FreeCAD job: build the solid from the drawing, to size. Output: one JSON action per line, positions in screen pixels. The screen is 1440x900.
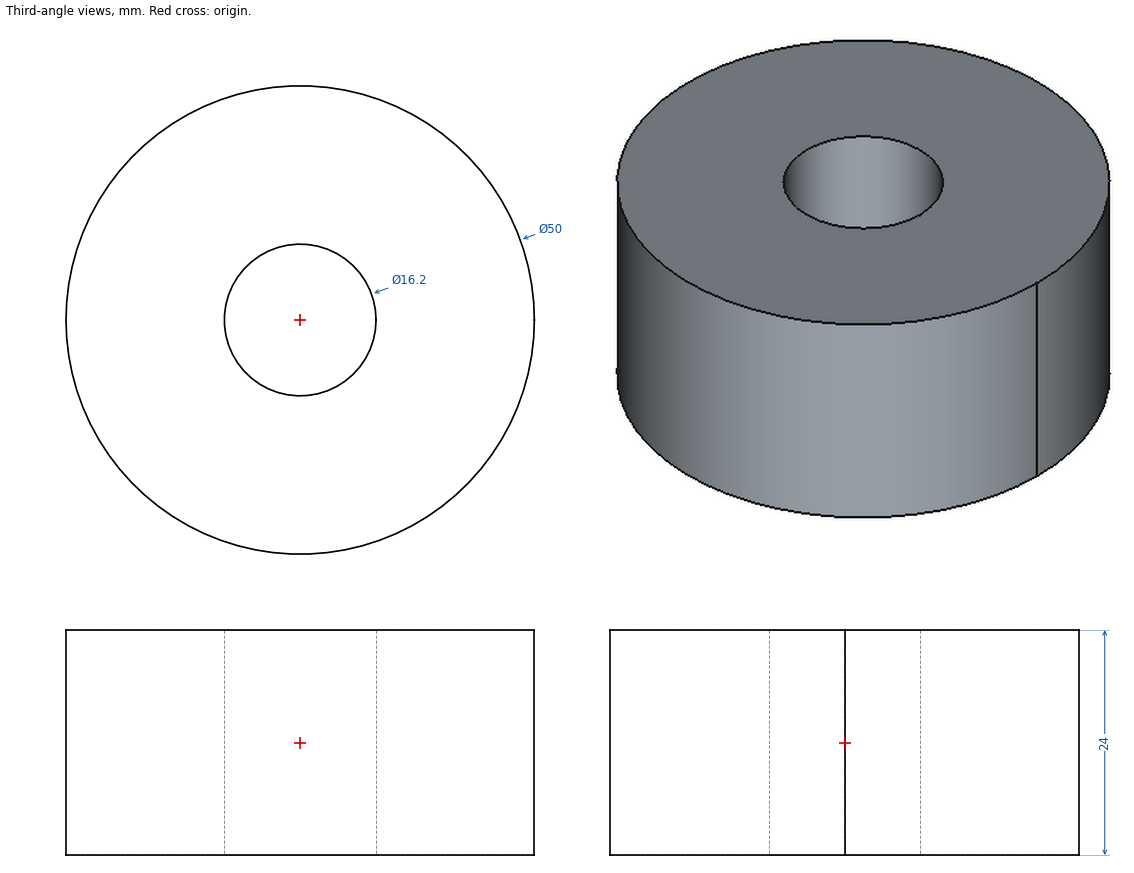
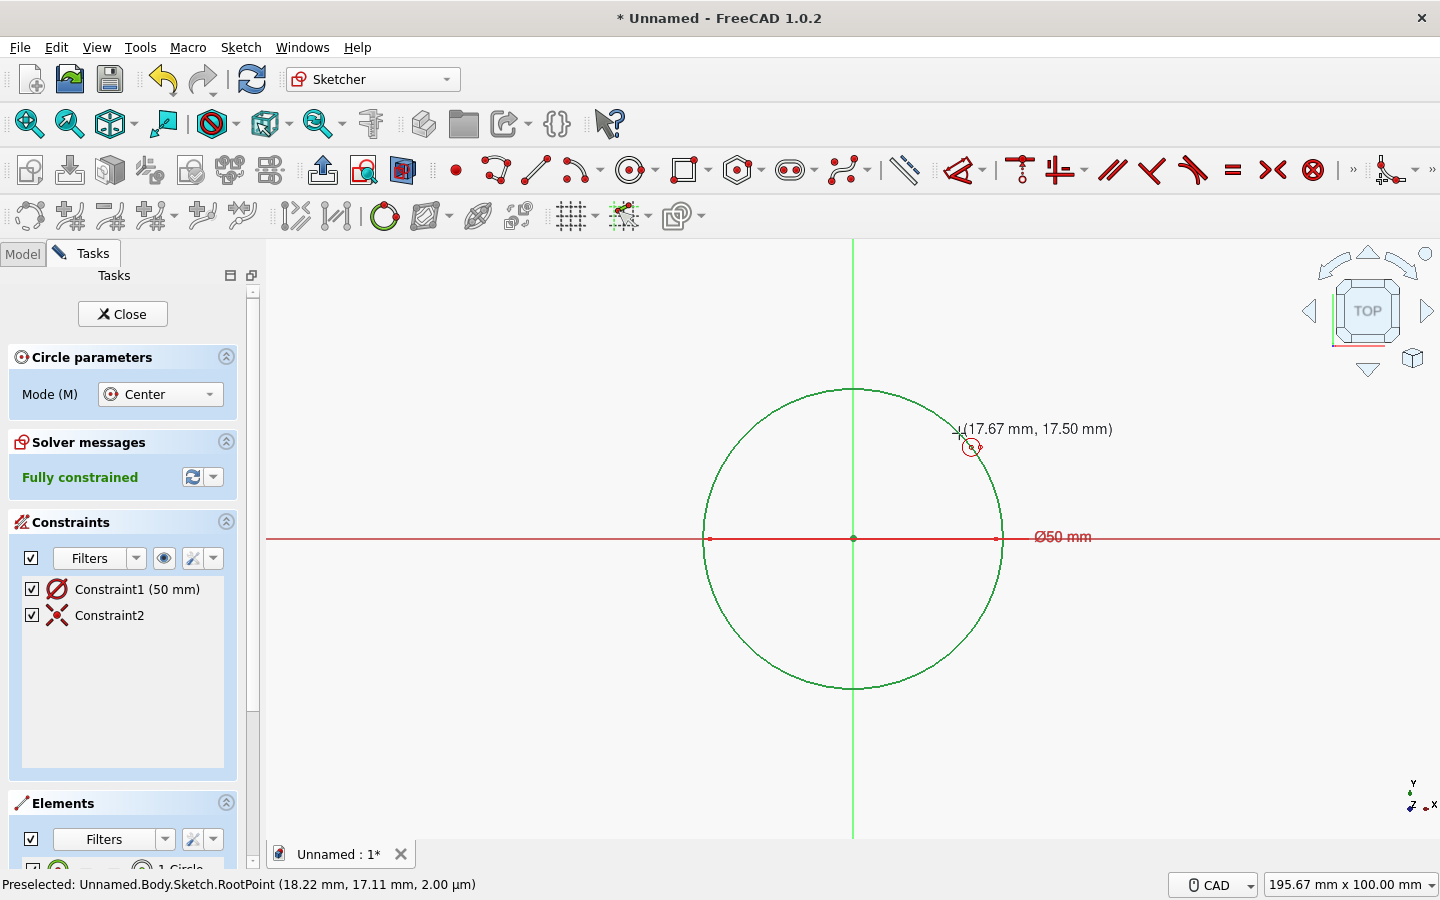
{"action": "left_click", "coordinate": [853, 539]}
{"action": "mouse_move", "coordinate": [887, 505]}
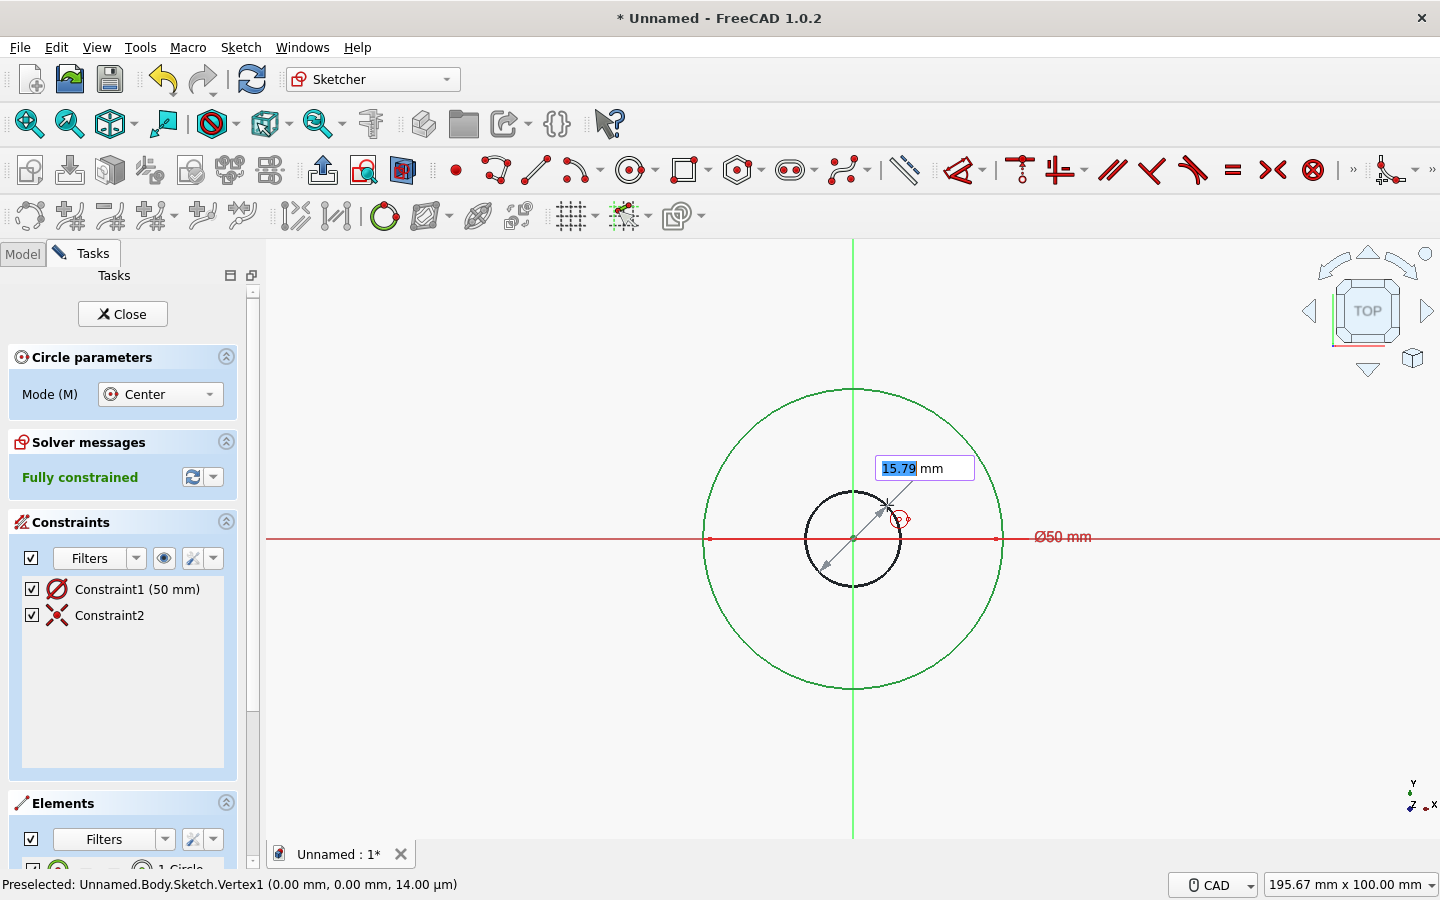
{"action": "type", "text": "16.2"}
{"action": "key", "text": "Return"}
{"action": "key", "text": "Escape"}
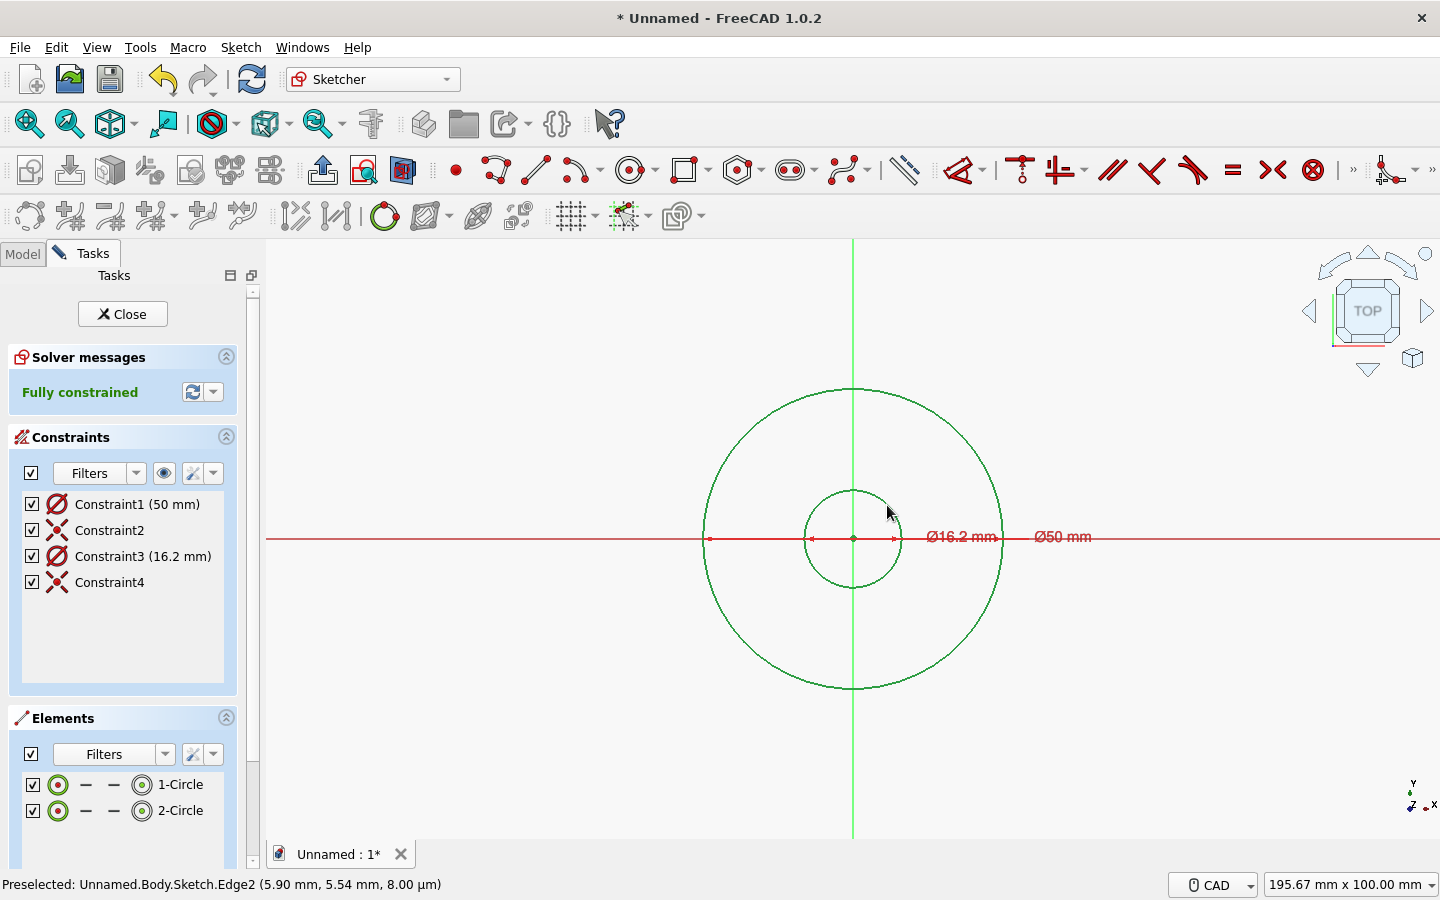
{"action": "left_click", "coordinate": [123, 314]}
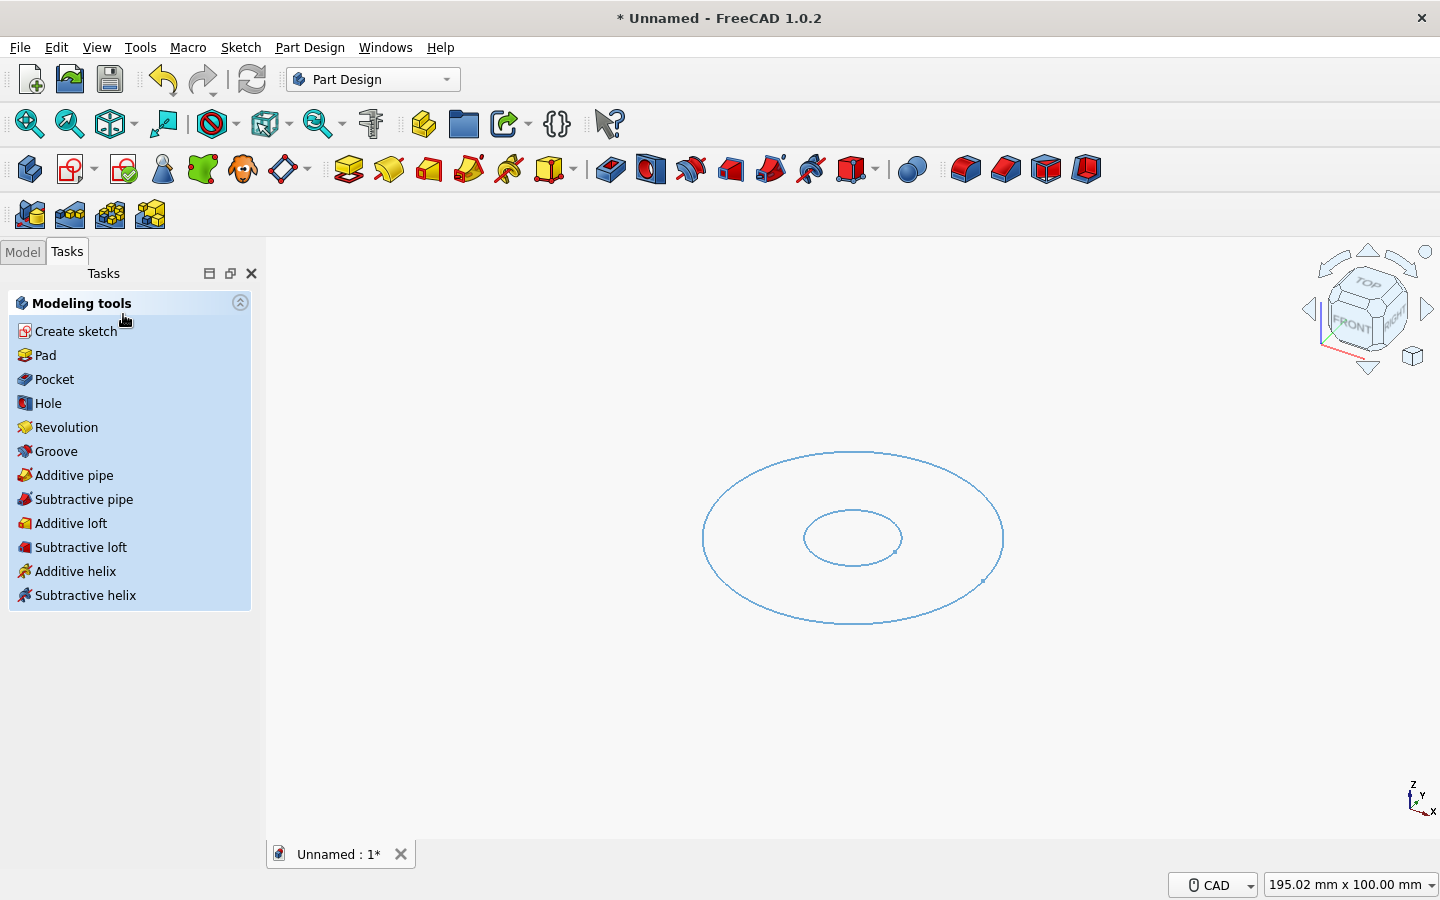
{"action": "left_click", "coordinate": [350, 170]}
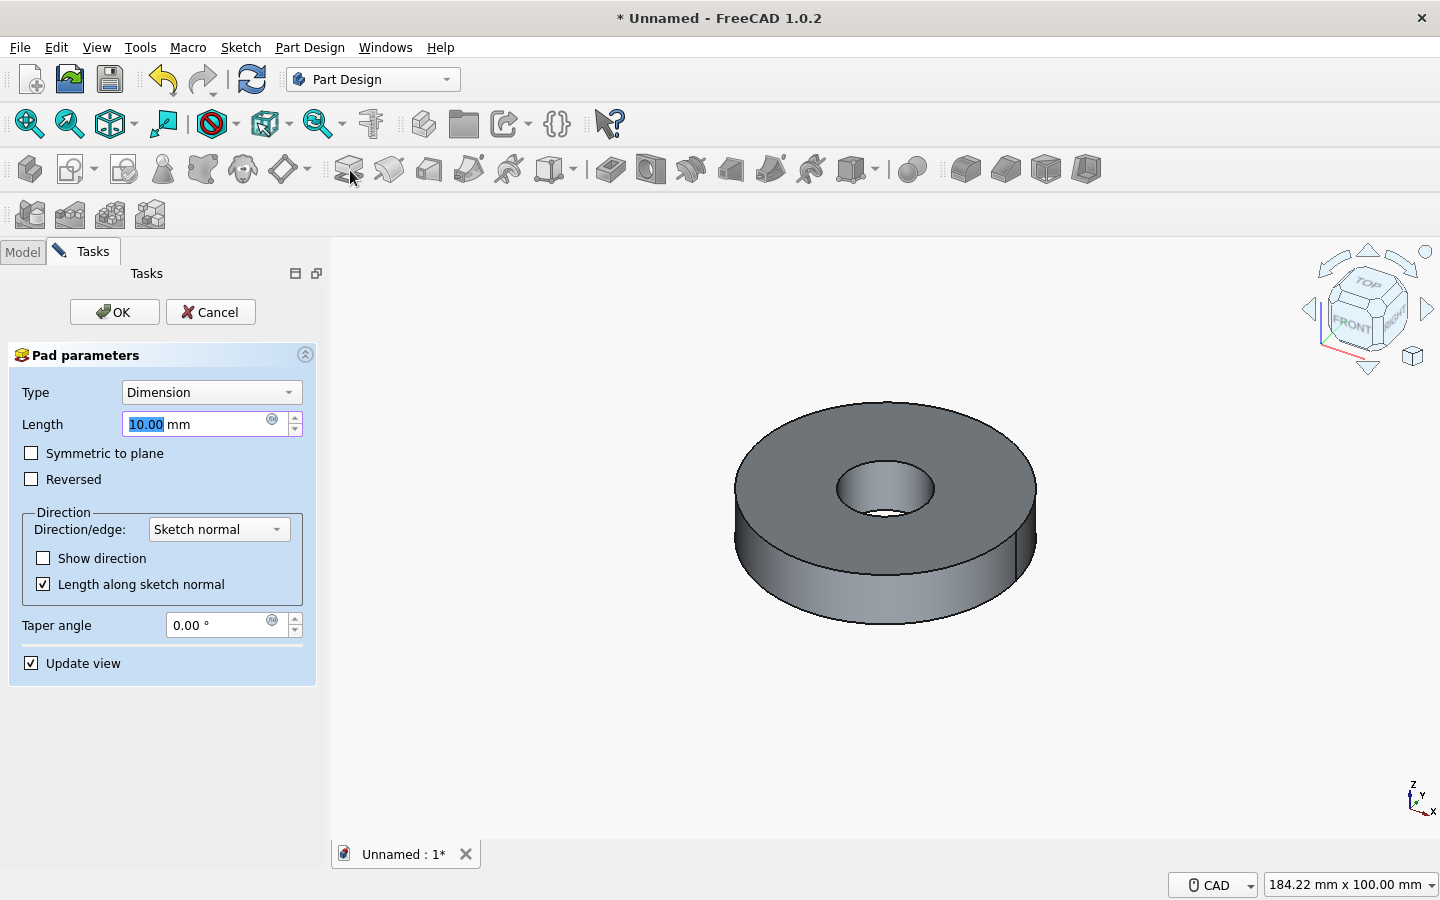
{"action": "type", "text": "24"}
{"action": "key", "text": "Tab"}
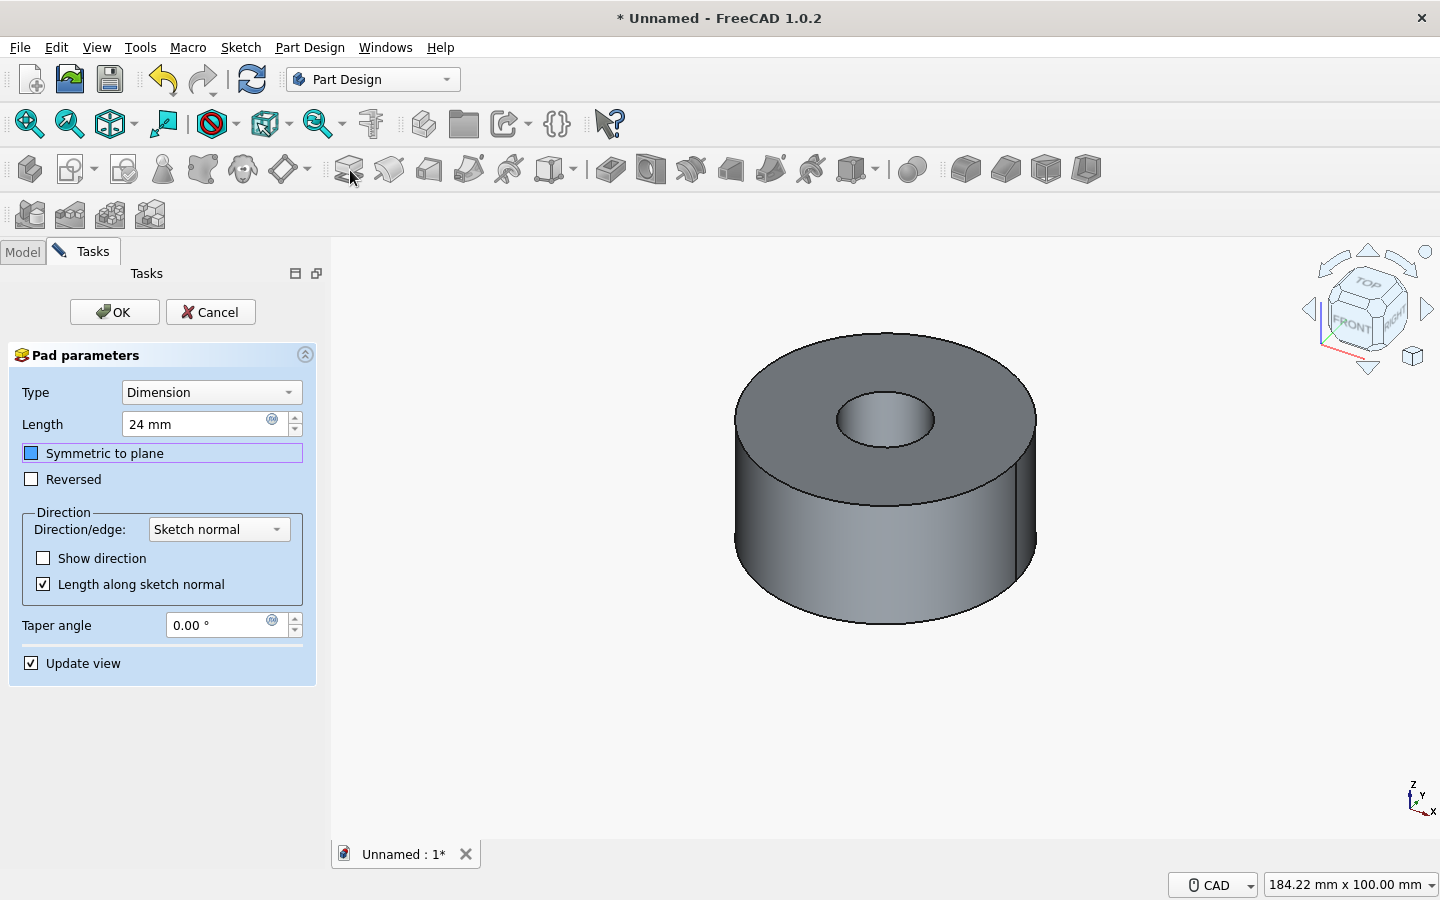
{"action": "left_click", "coordinate": [30, 453]}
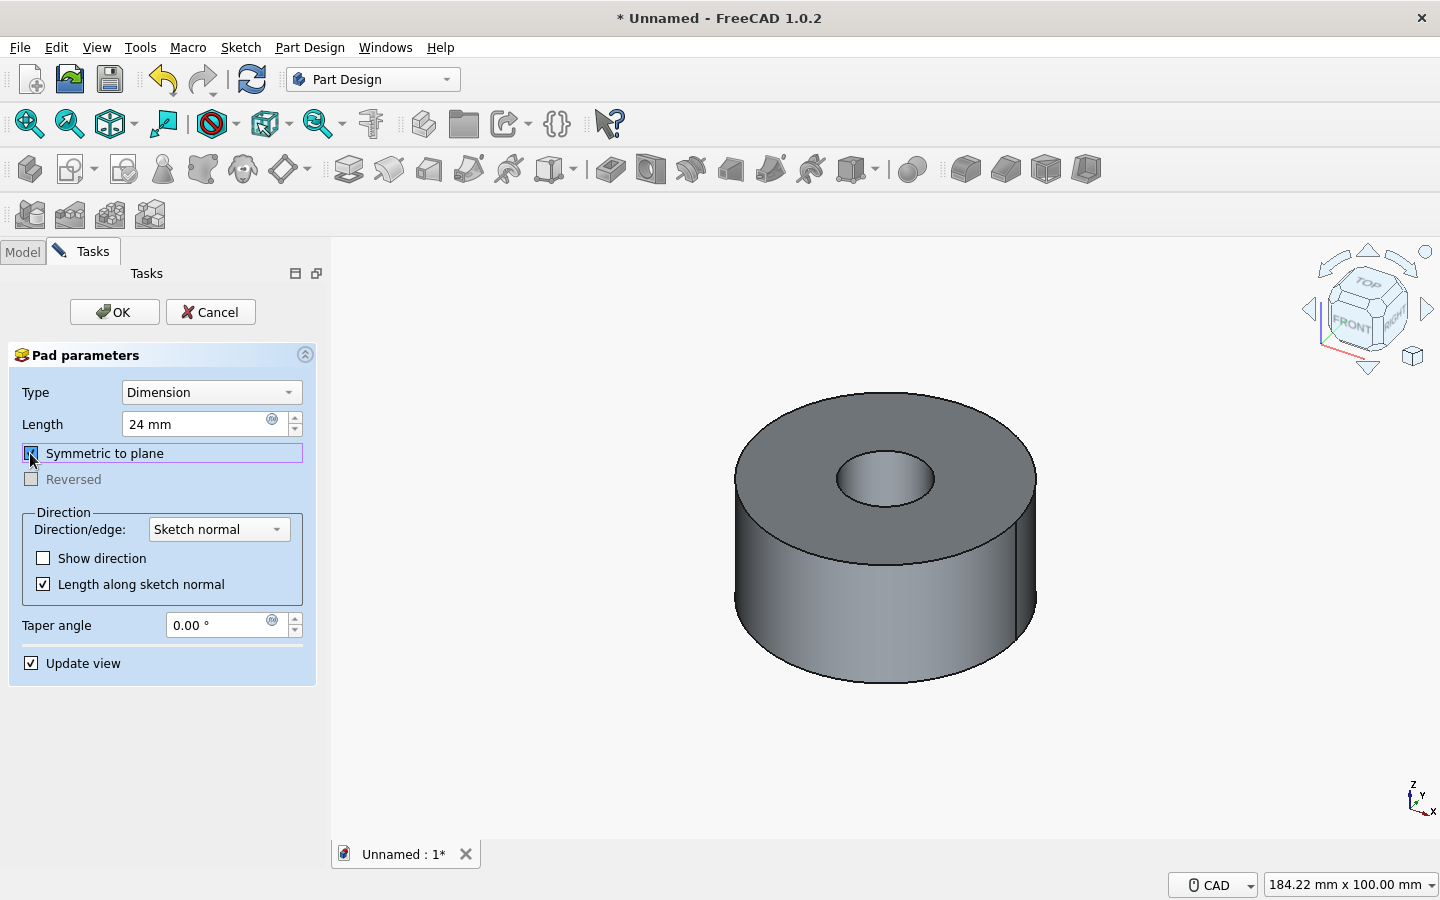
{"action": "left_click", "coordinate": [115, 312]}